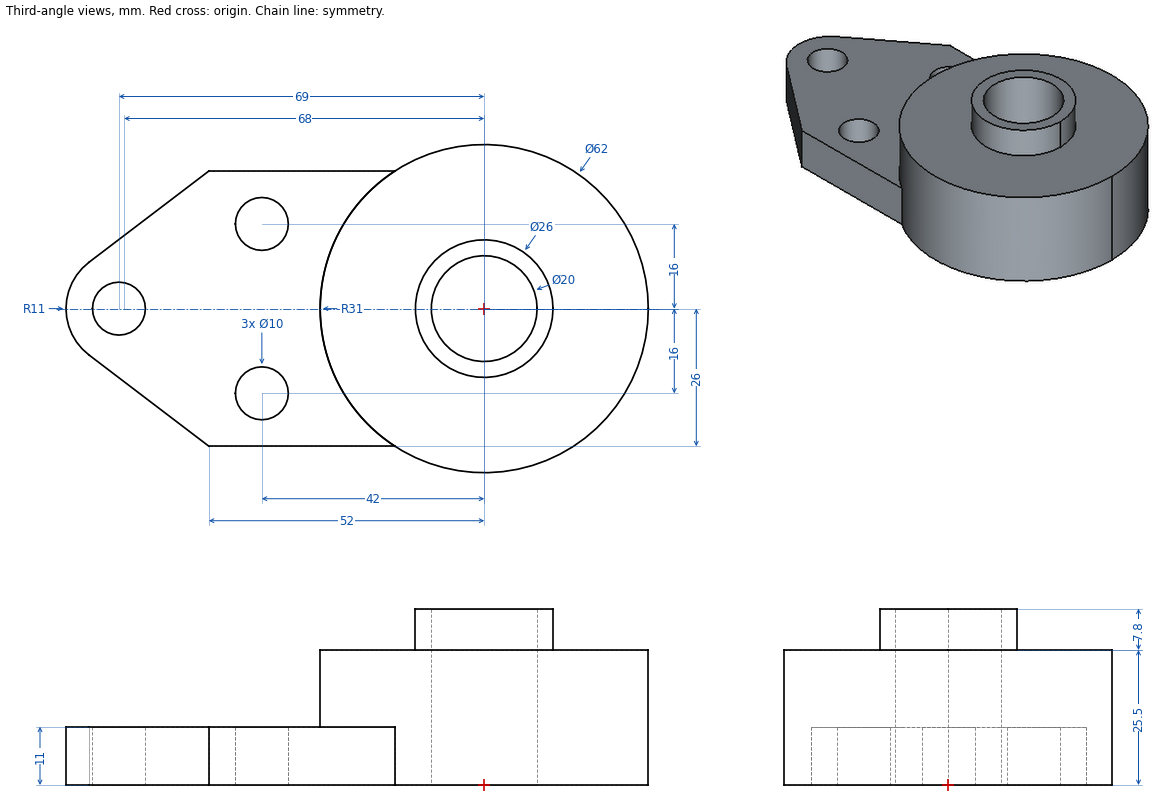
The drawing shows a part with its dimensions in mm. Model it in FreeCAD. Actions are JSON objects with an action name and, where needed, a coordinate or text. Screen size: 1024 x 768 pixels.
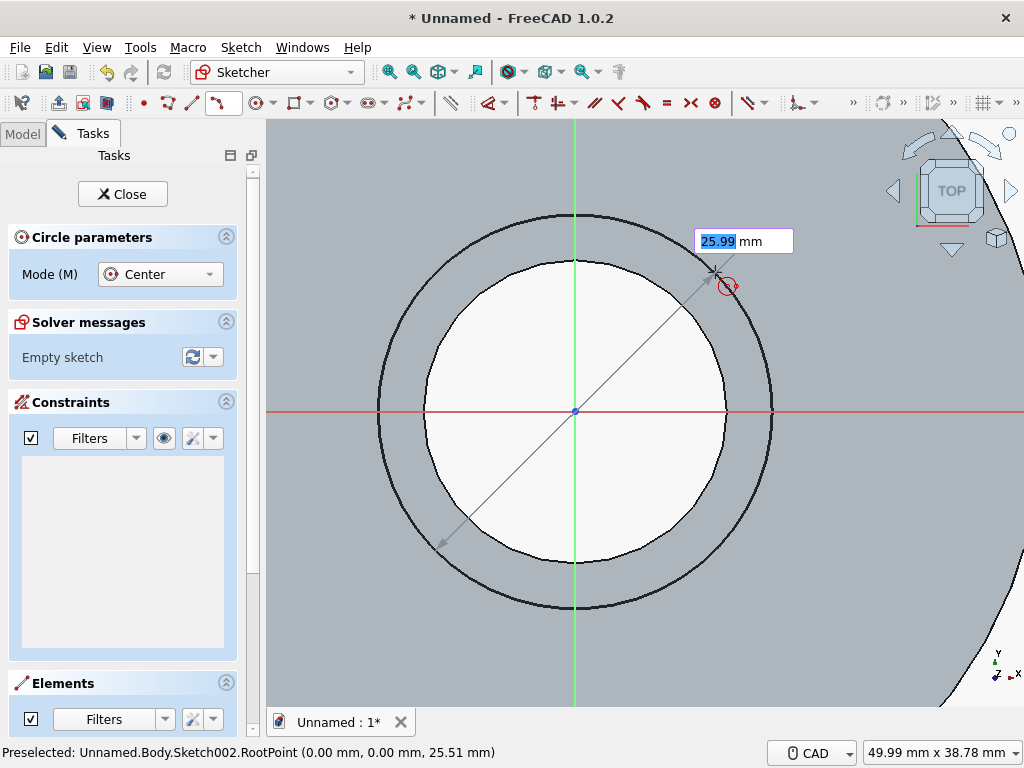
{"action": "type", "text": "26"}
{"action": "key", "text": "Return"}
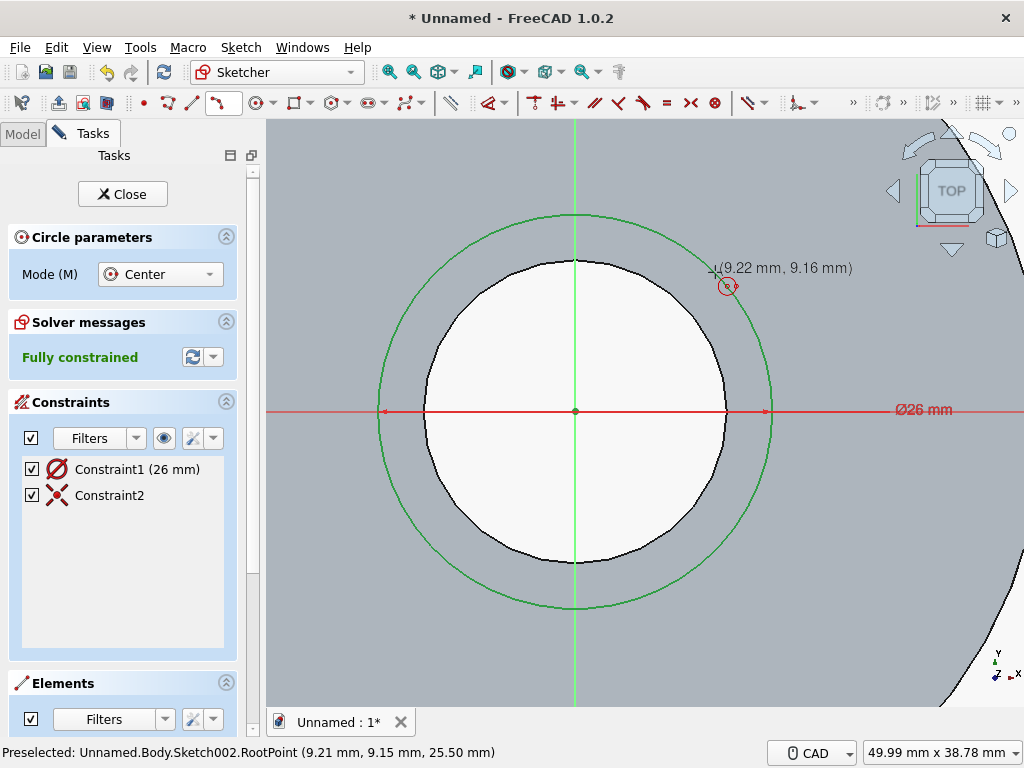
{"action": "left_click", "coordinate": [575, 412]}
{"action": "mouse_move", "coordinate": [682, 305]}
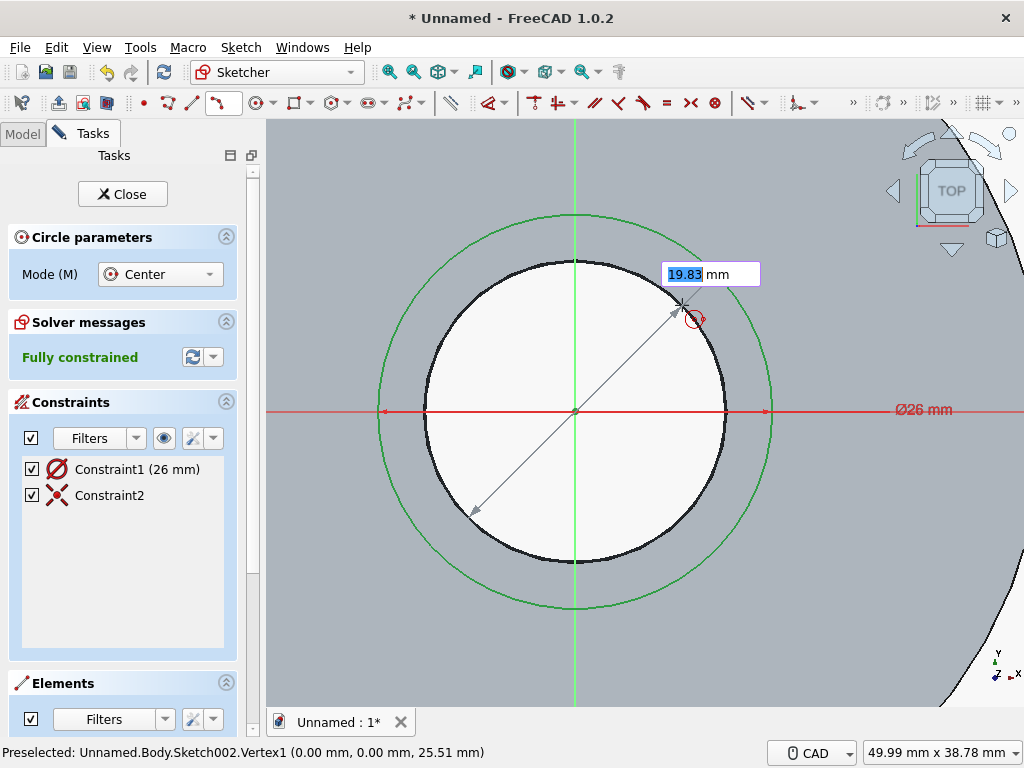
{"action": "type", "text": "20"}
{"action": "key", "text": "Return"}
{"action": "key", "text": "Escape"}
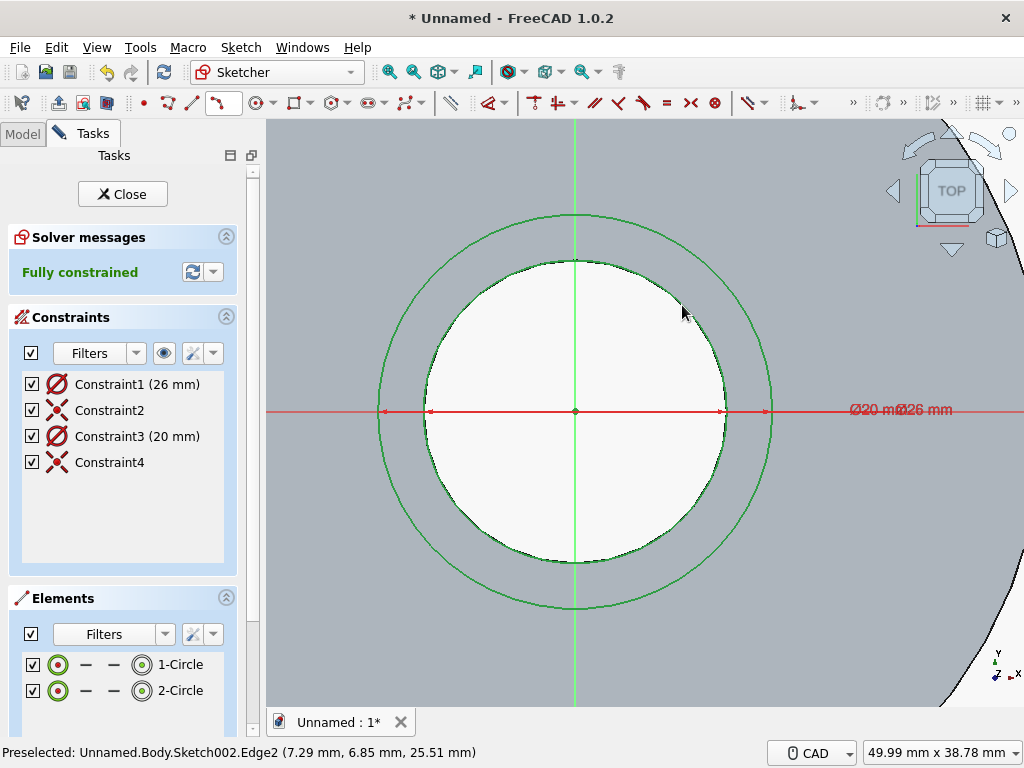
{"action": "left_click", "coordinate": [123, 194]}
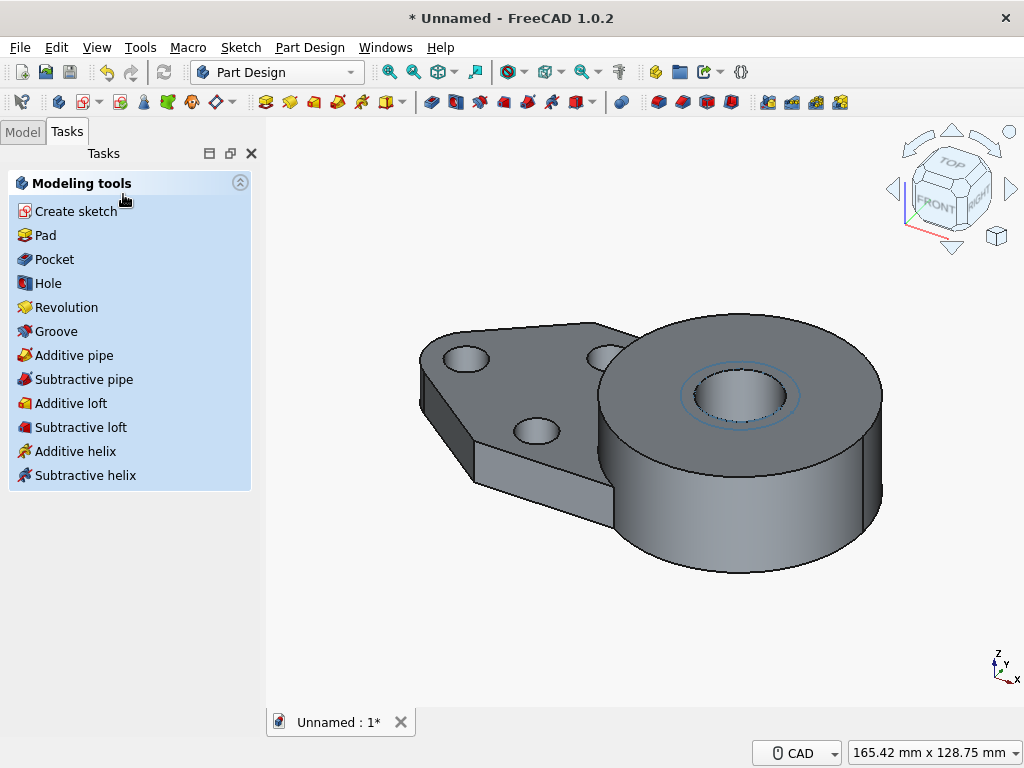
{"action": "left_click", "coordinate": [266, 102]}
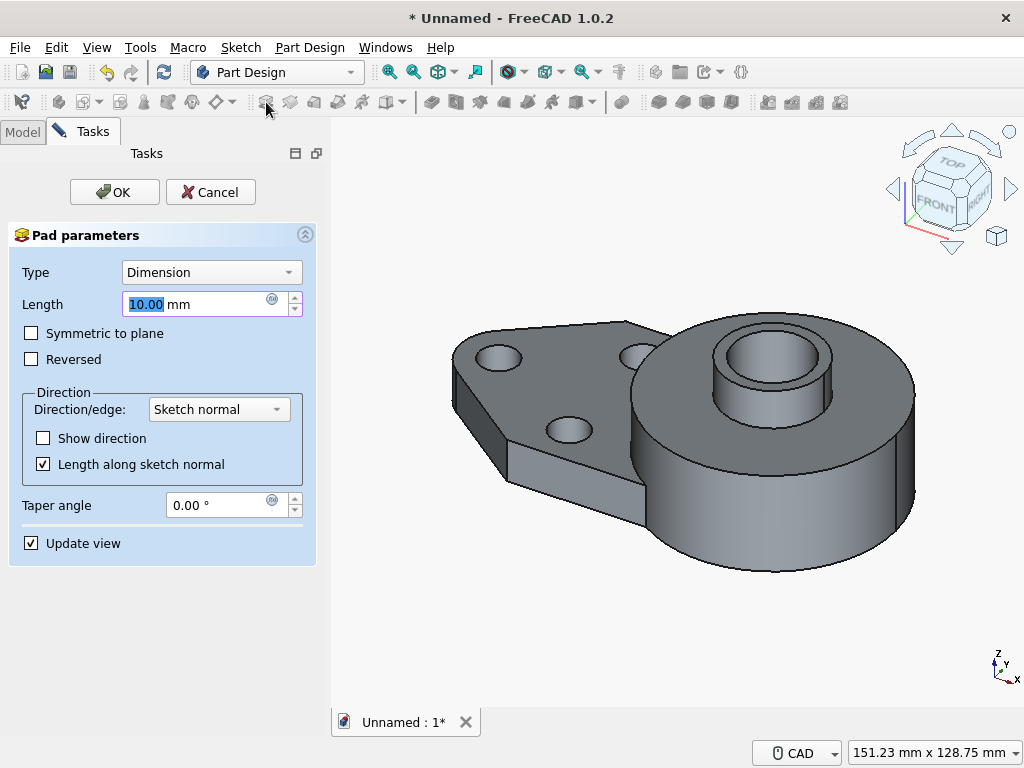
{"action": "type", "text": "7.8"}
{"action": "key", "text": "Tab"}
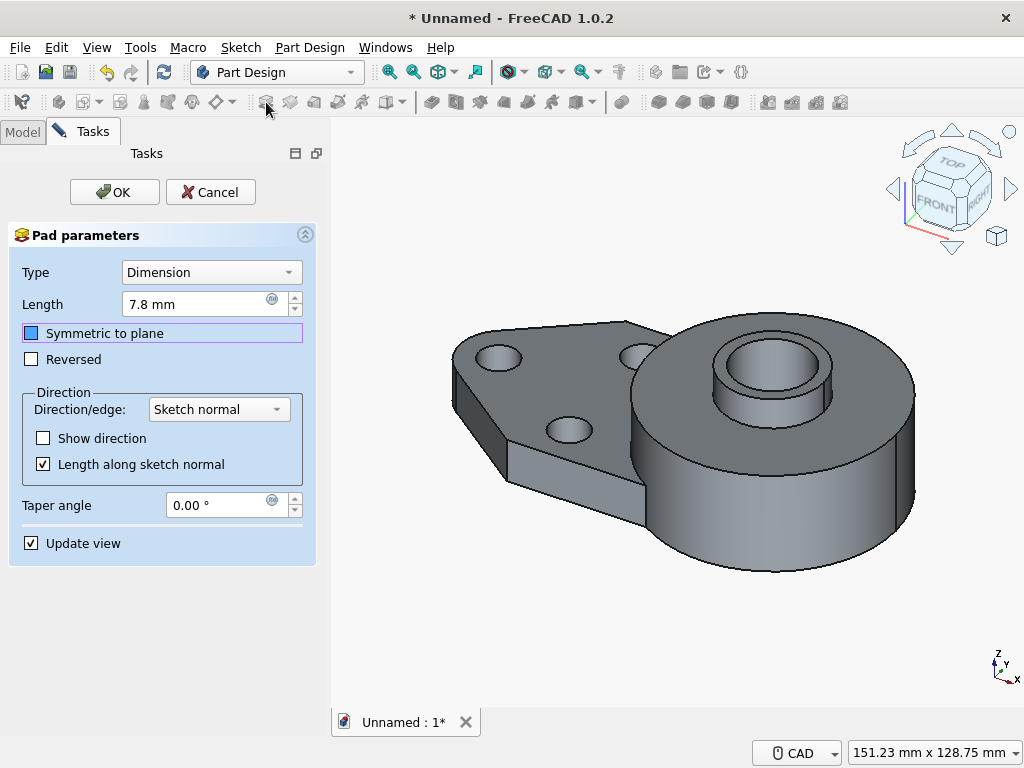
{"action": "left_click", "coordinate": [115, 192]}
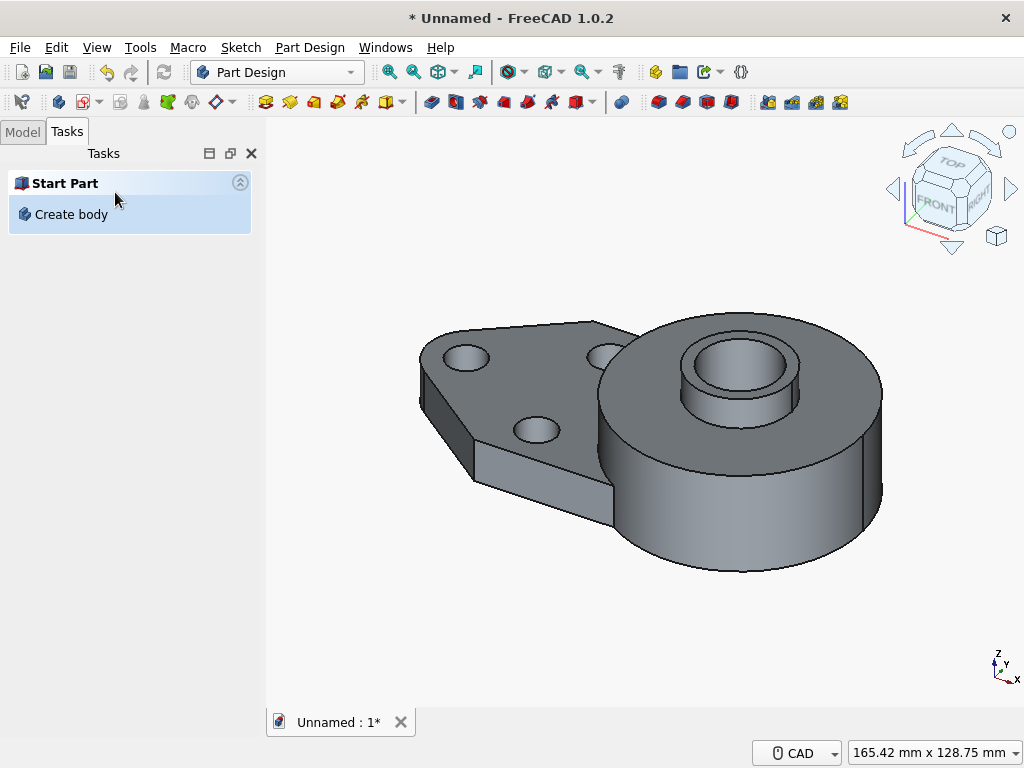
{"action": "key", "text": "0"}